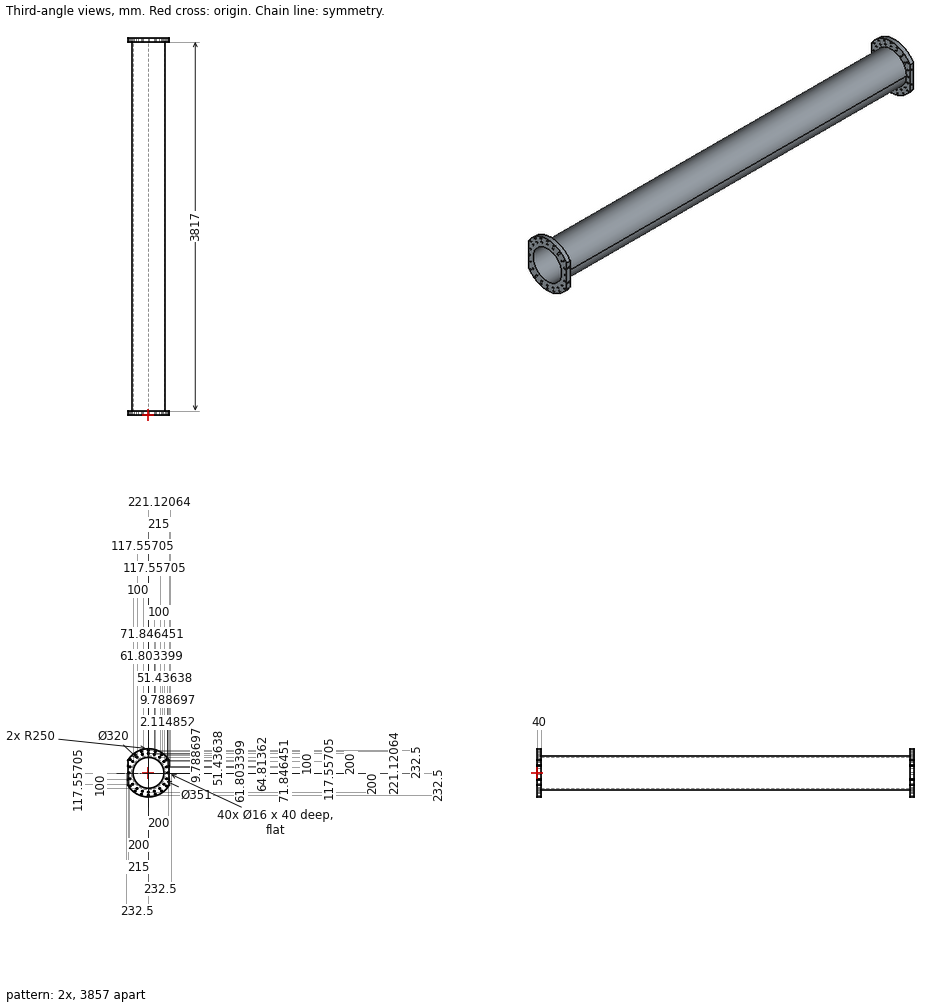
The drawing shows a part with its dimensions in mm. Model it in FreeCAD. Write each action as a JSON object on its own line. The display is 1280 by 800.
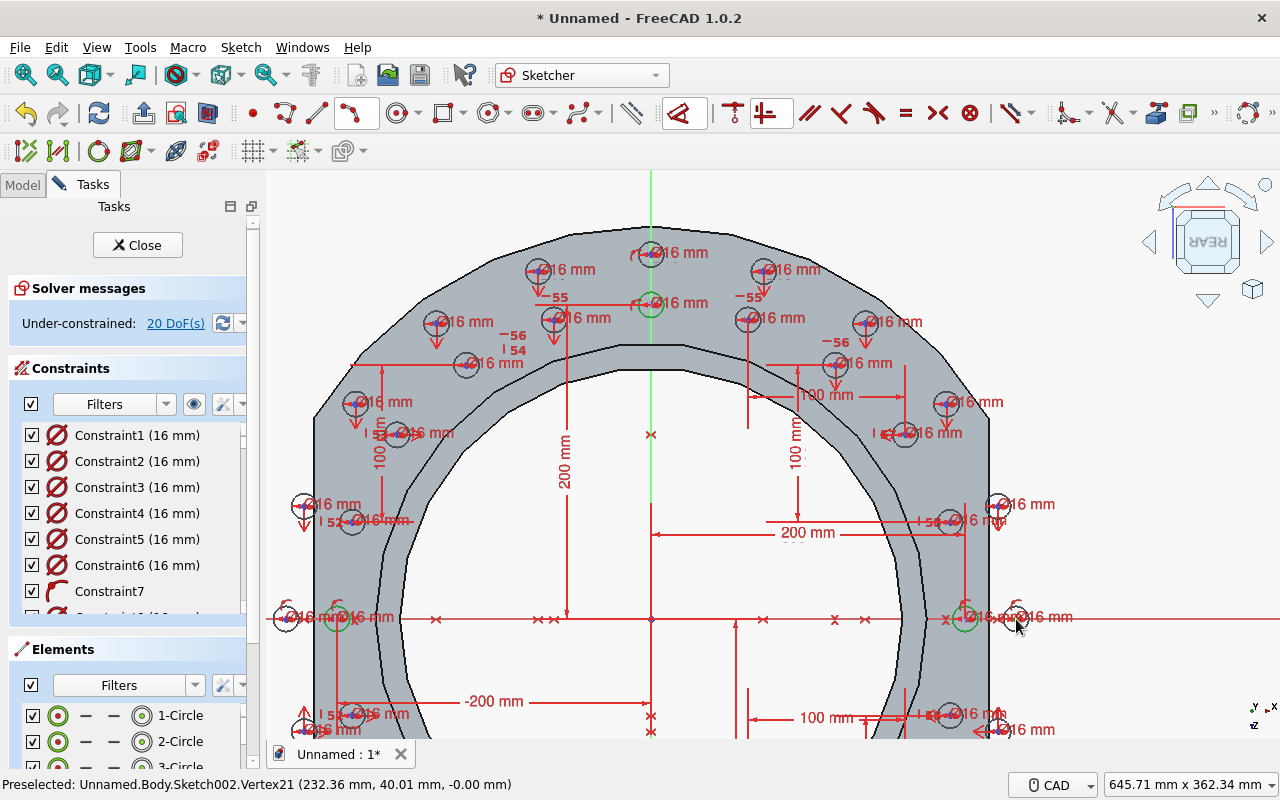
{"action": "key", "text": "l"}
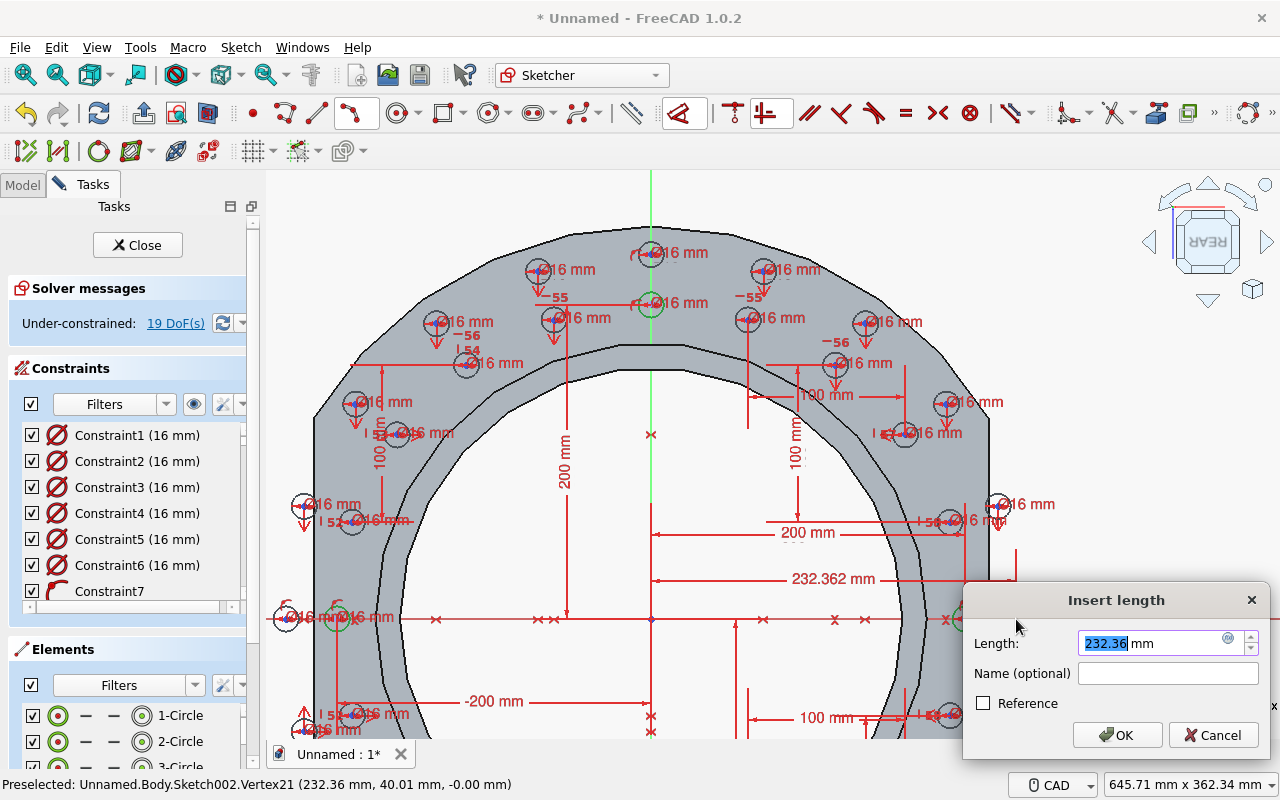
{"action": "type", "text": "232.5"}
{"action": "key", "text": "Return"}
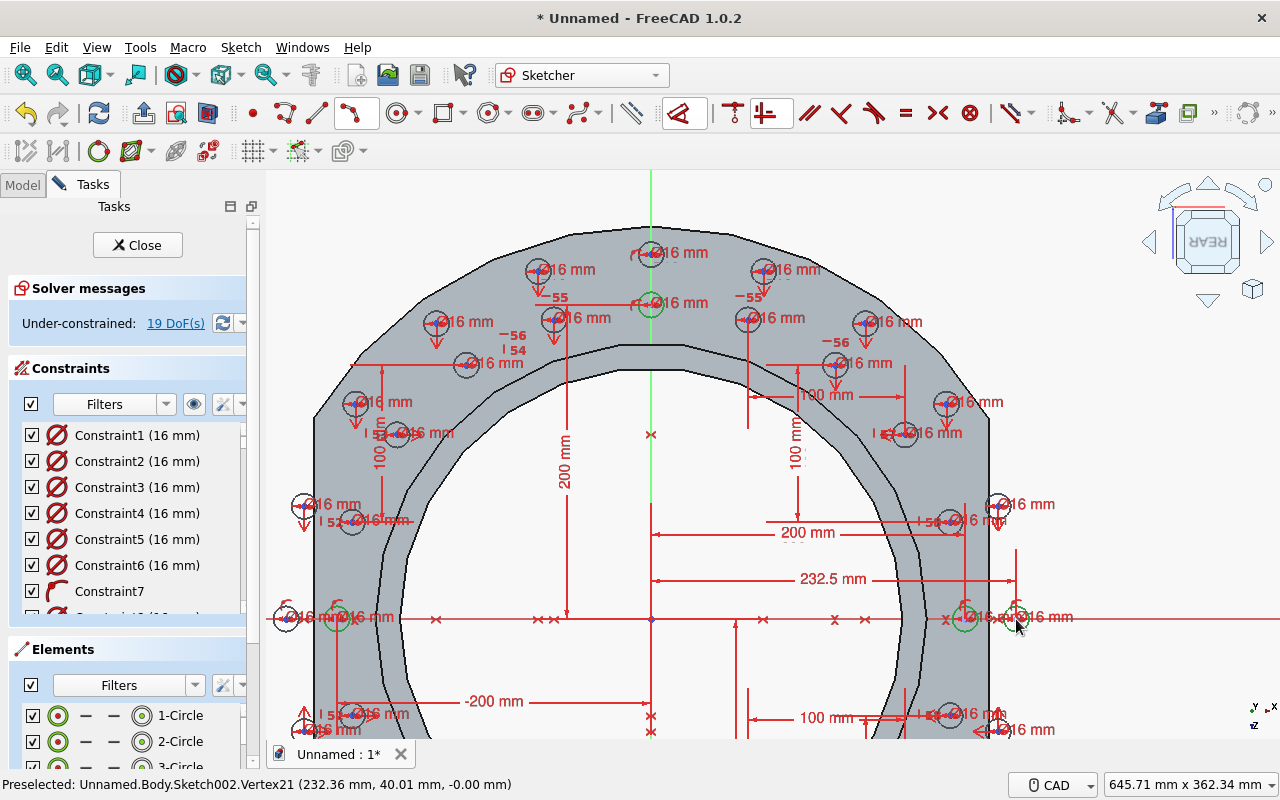
{"action": "scroll", "coordinate": [748, 320], "scroll_direction": "down", "scroll_amount": 4}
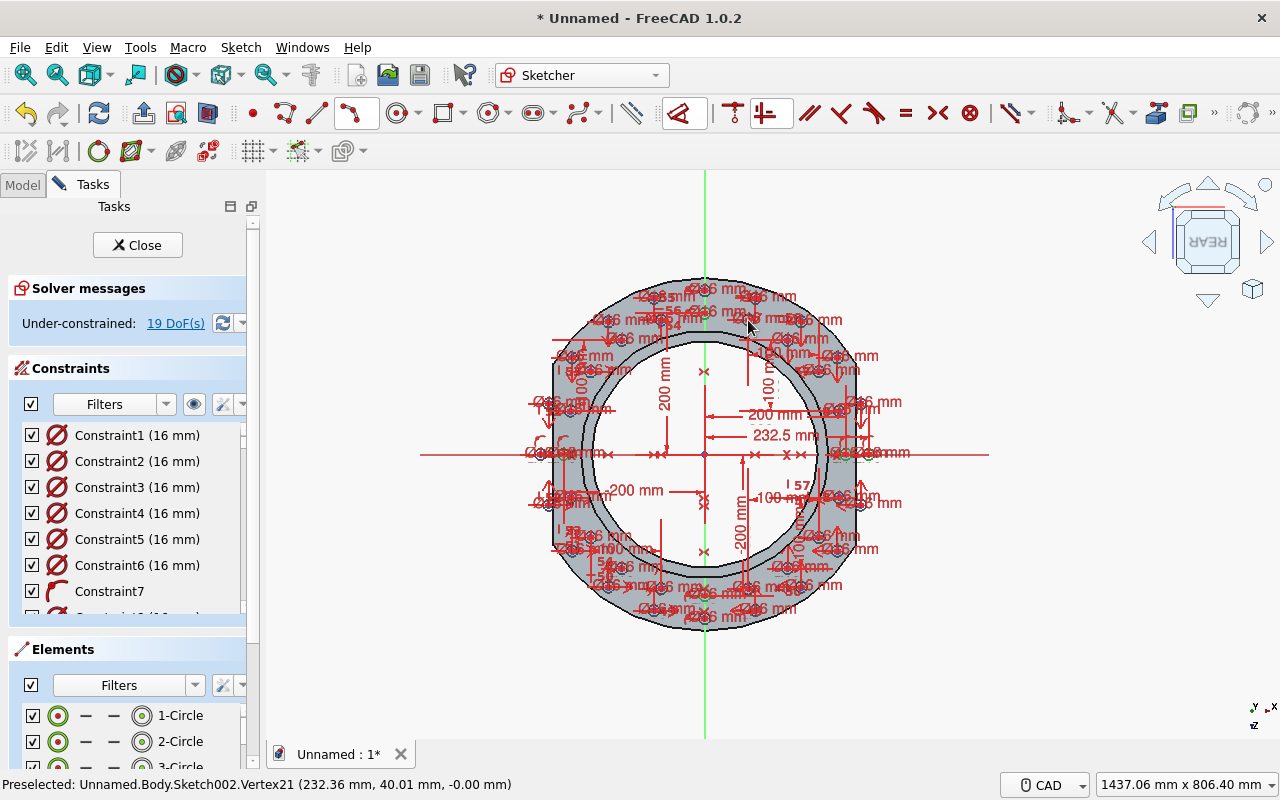
{"action": "left_click", "coordinate": [705, 619]}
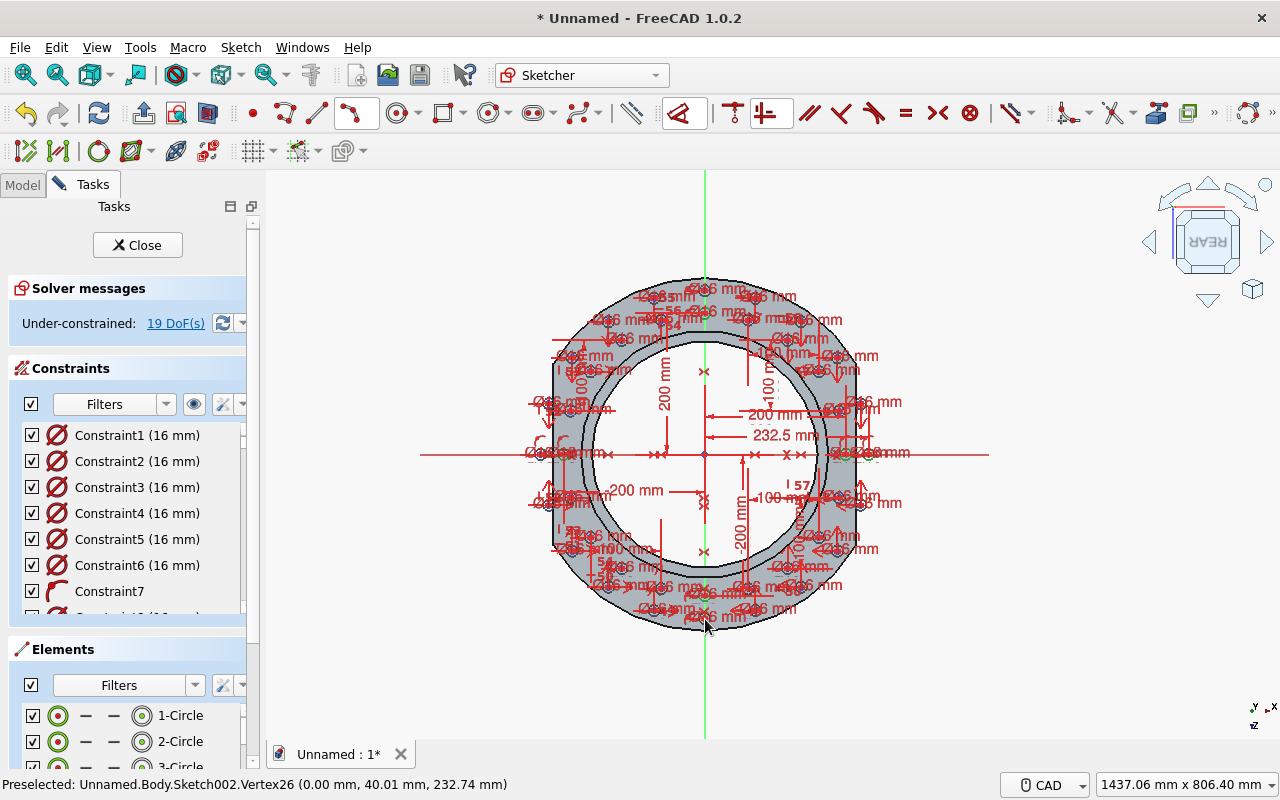
{"action": "left_click", "coordinate": [702, 114]}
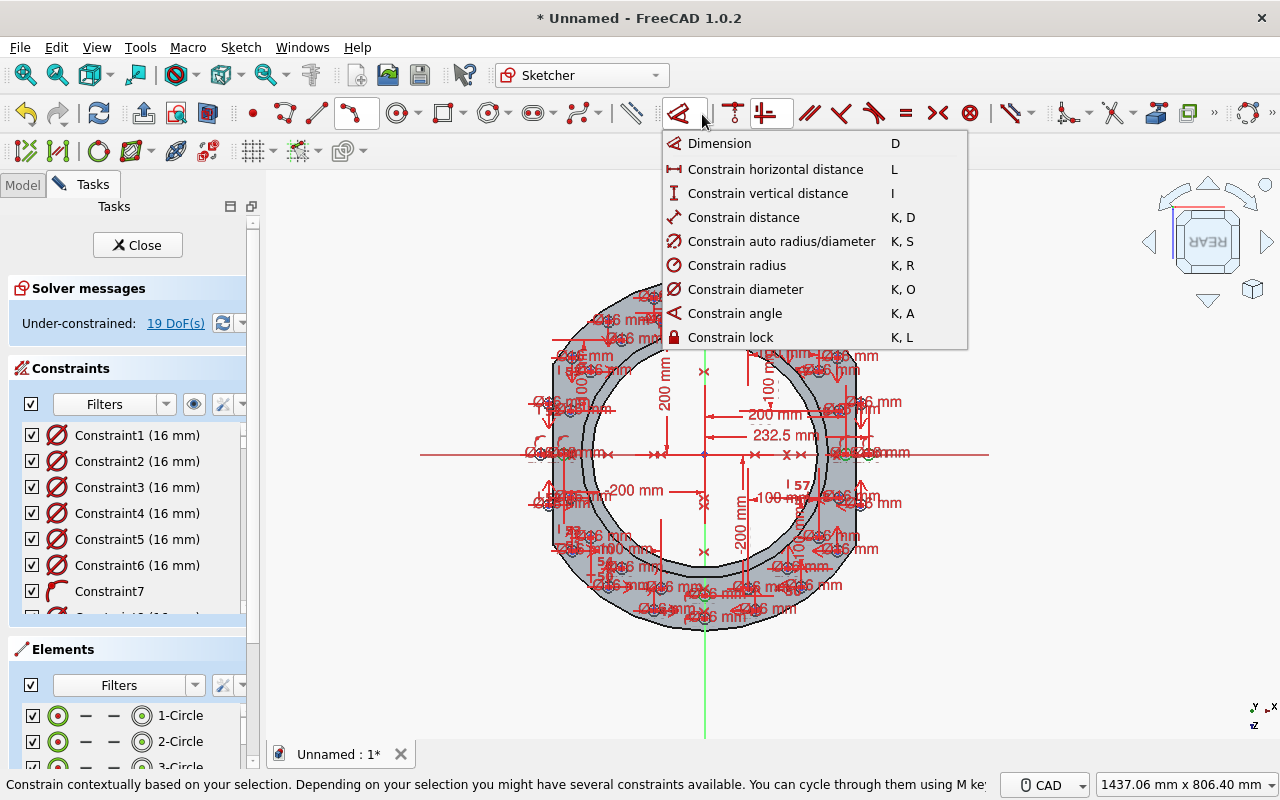
{"action": "left_click", "coordinate": [815, 193]}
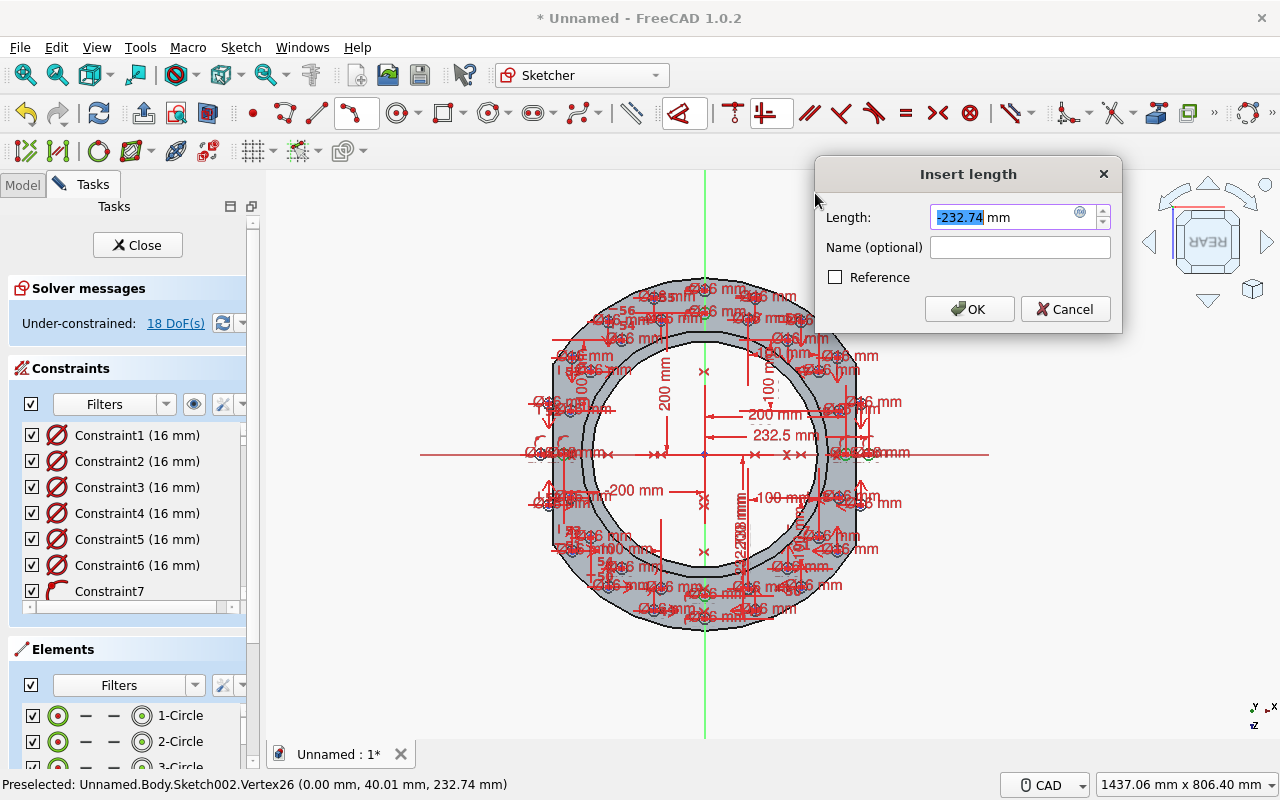
{"action": "type", "text": "-232.5"}
{"action": "key", "text": "Return"}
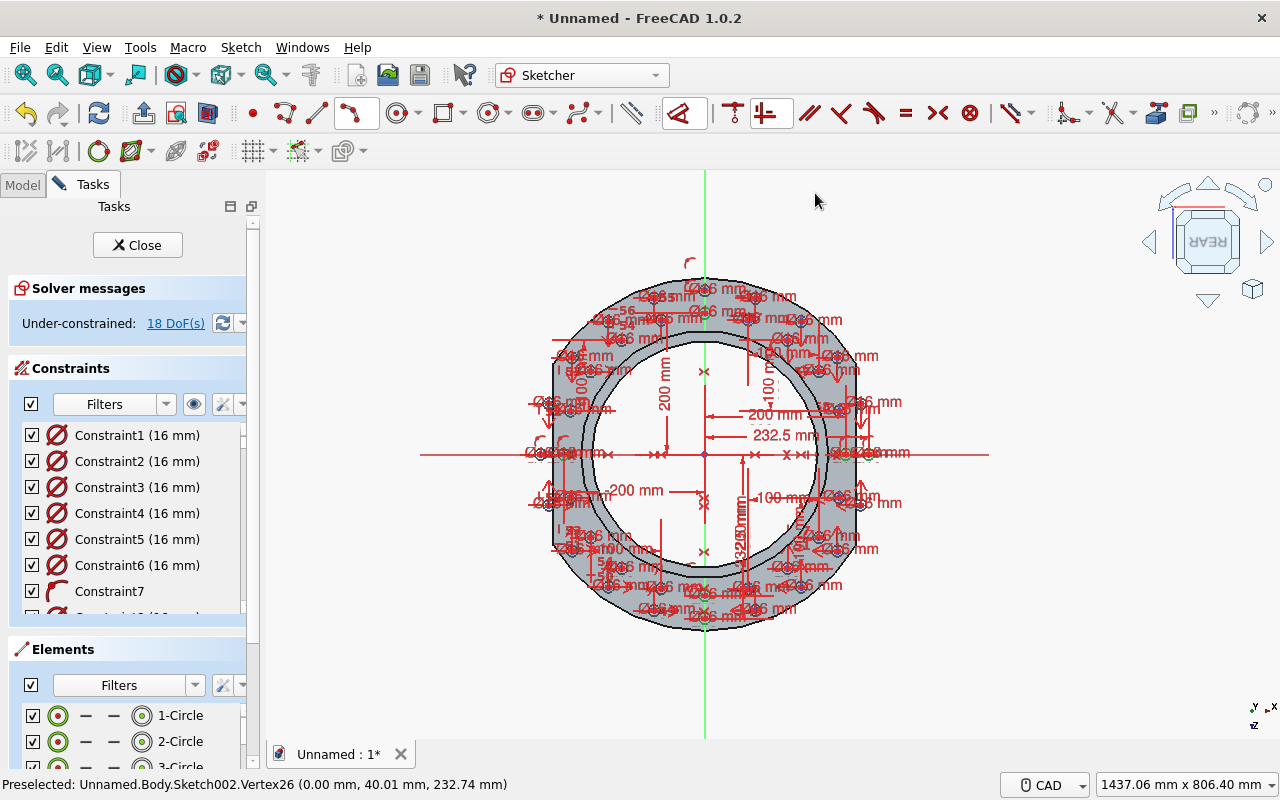
{"action": "left_click", "coordinate": [541, 454]}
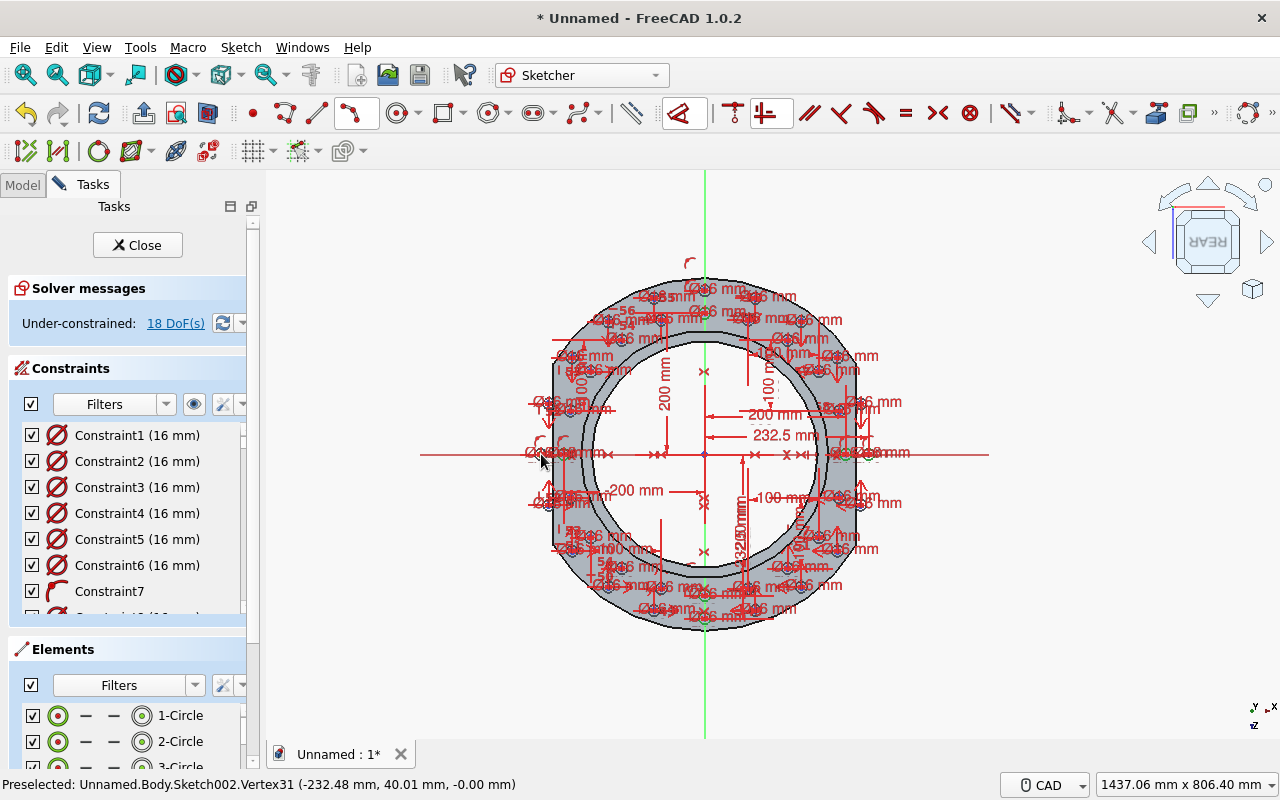
{"action": "key", "text": "l"}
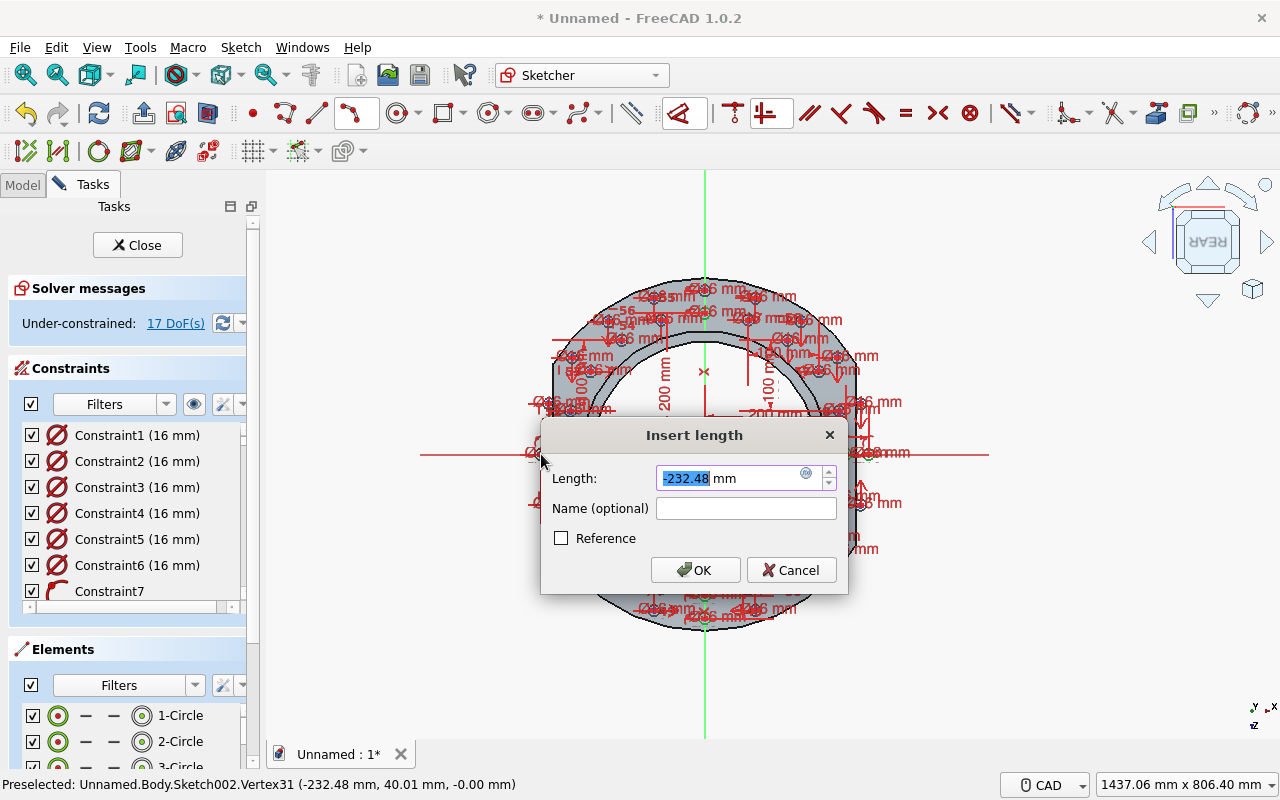
{"action": "type", "text": "-232.5"}
{"action": "key", "text": "Return"}